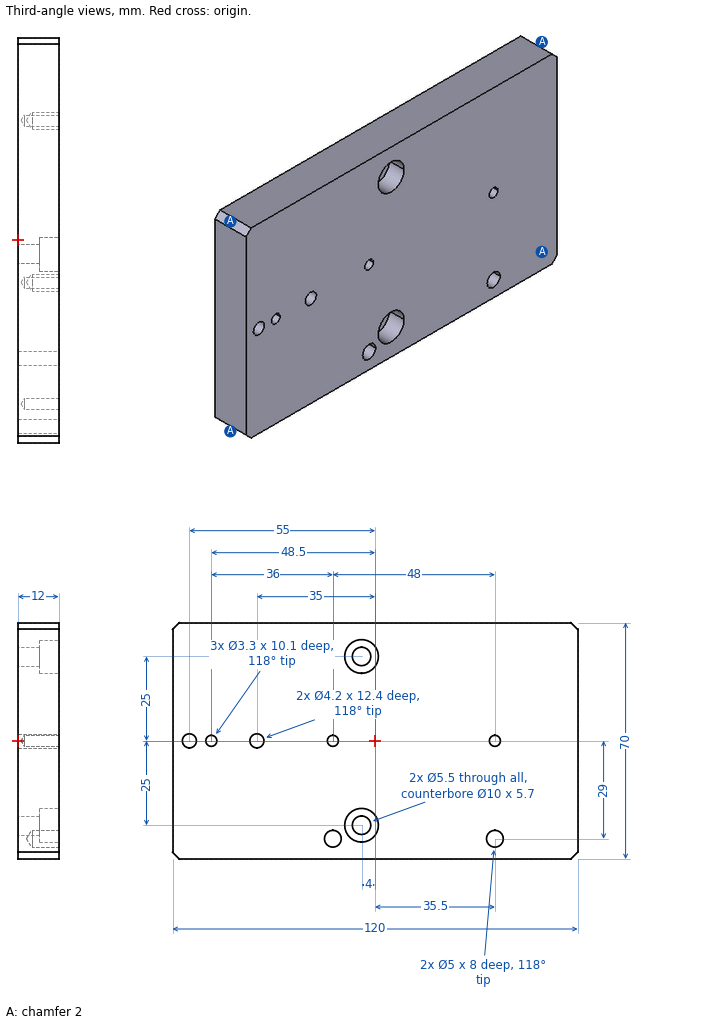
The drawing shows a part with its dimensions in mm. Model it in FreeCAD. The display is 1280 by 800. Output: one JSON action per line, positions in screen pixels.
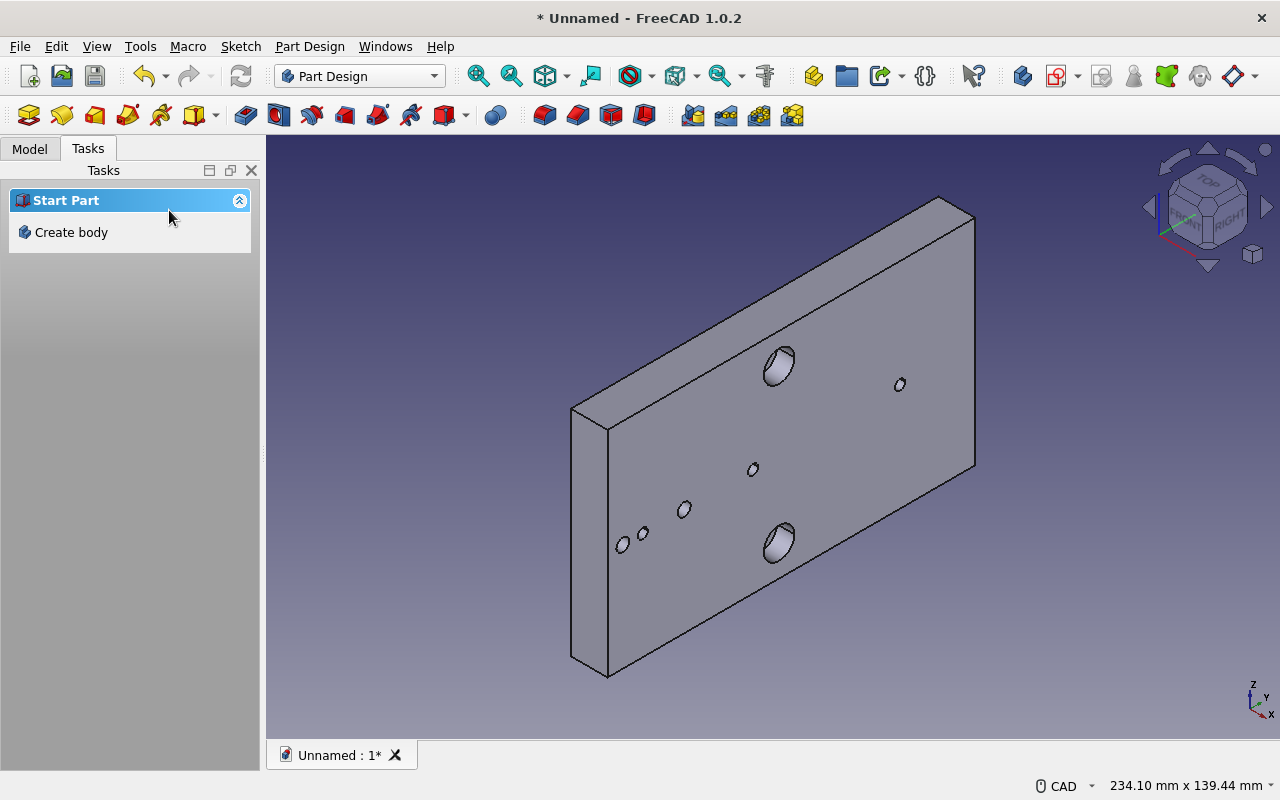
{"action": "left_click", "coordinate": [844, 452]}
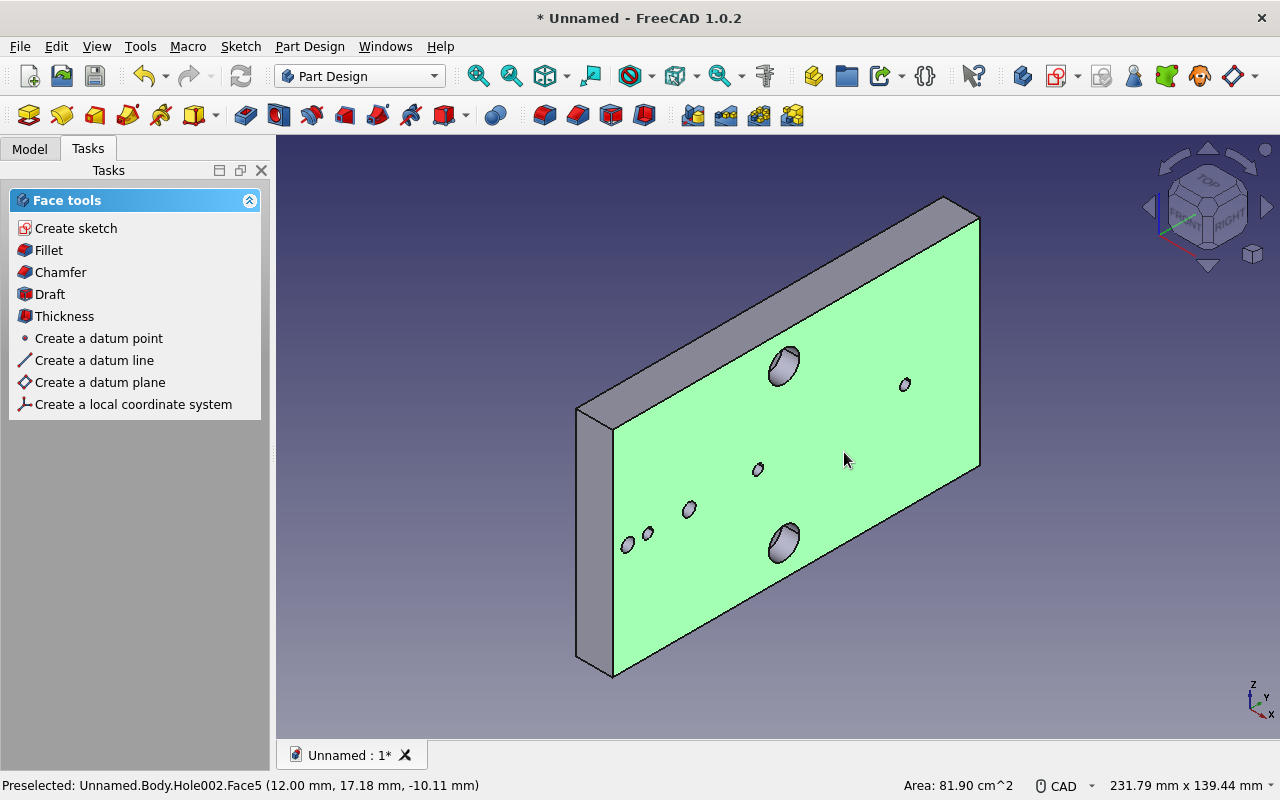
{"action": "left_click", "coordinate": [1056, 76]}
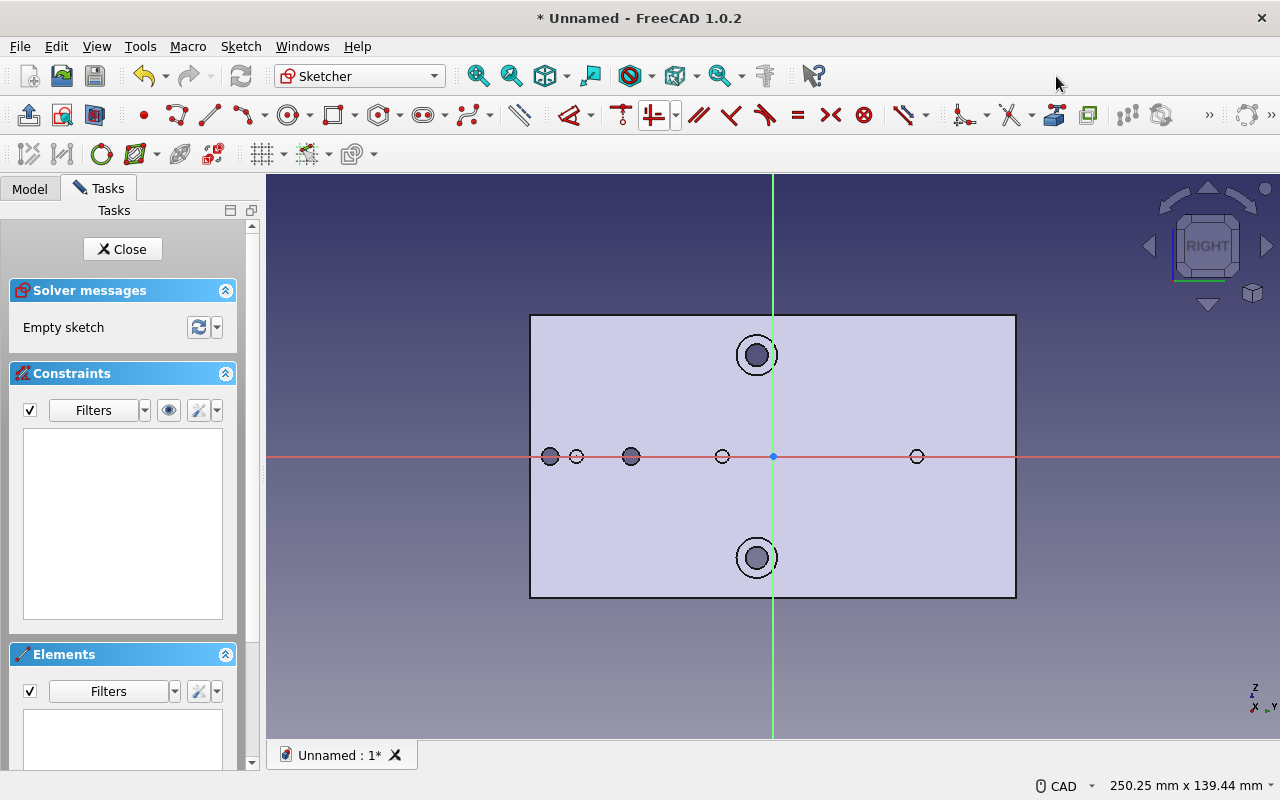
{"action": "scroll", "coordinate": [887, 557], "scroll_direction": "up", "scroll_amount": 5}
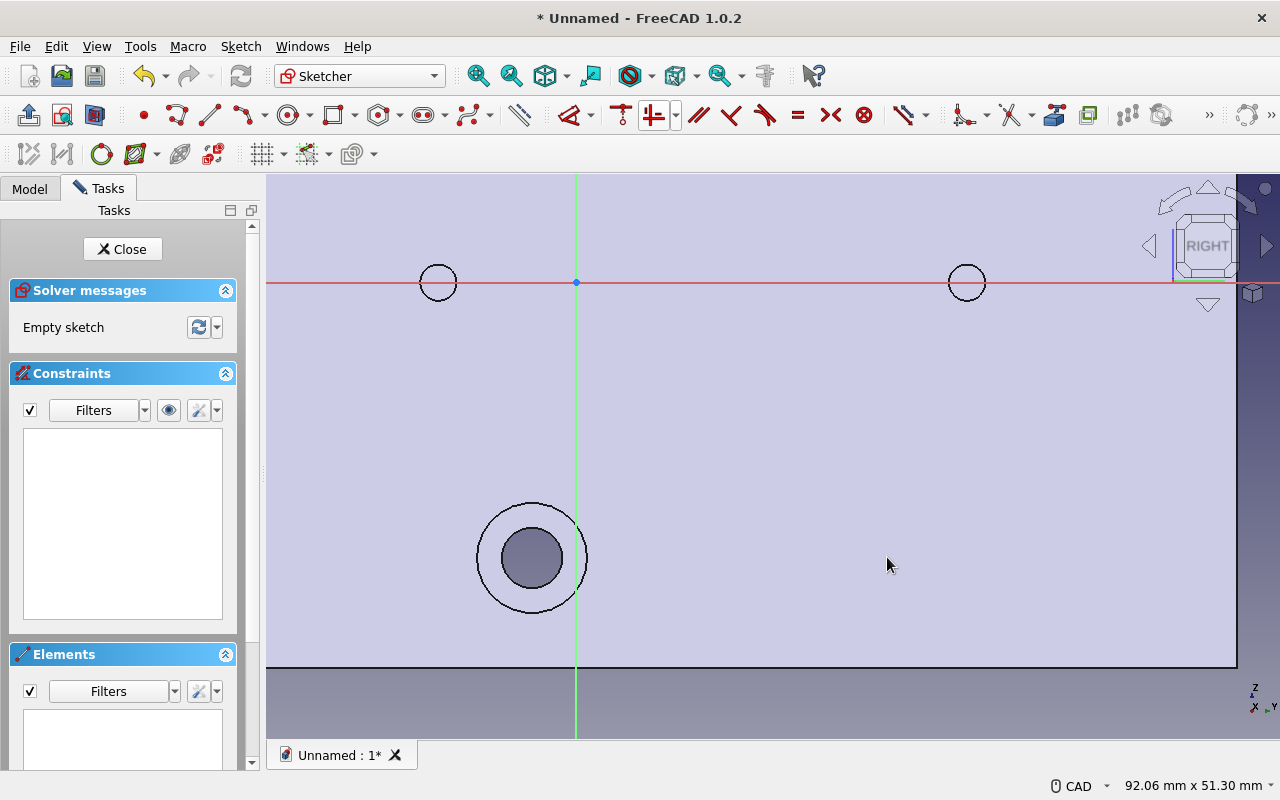
{"action": "left_click", "coordinate": [288, 116]}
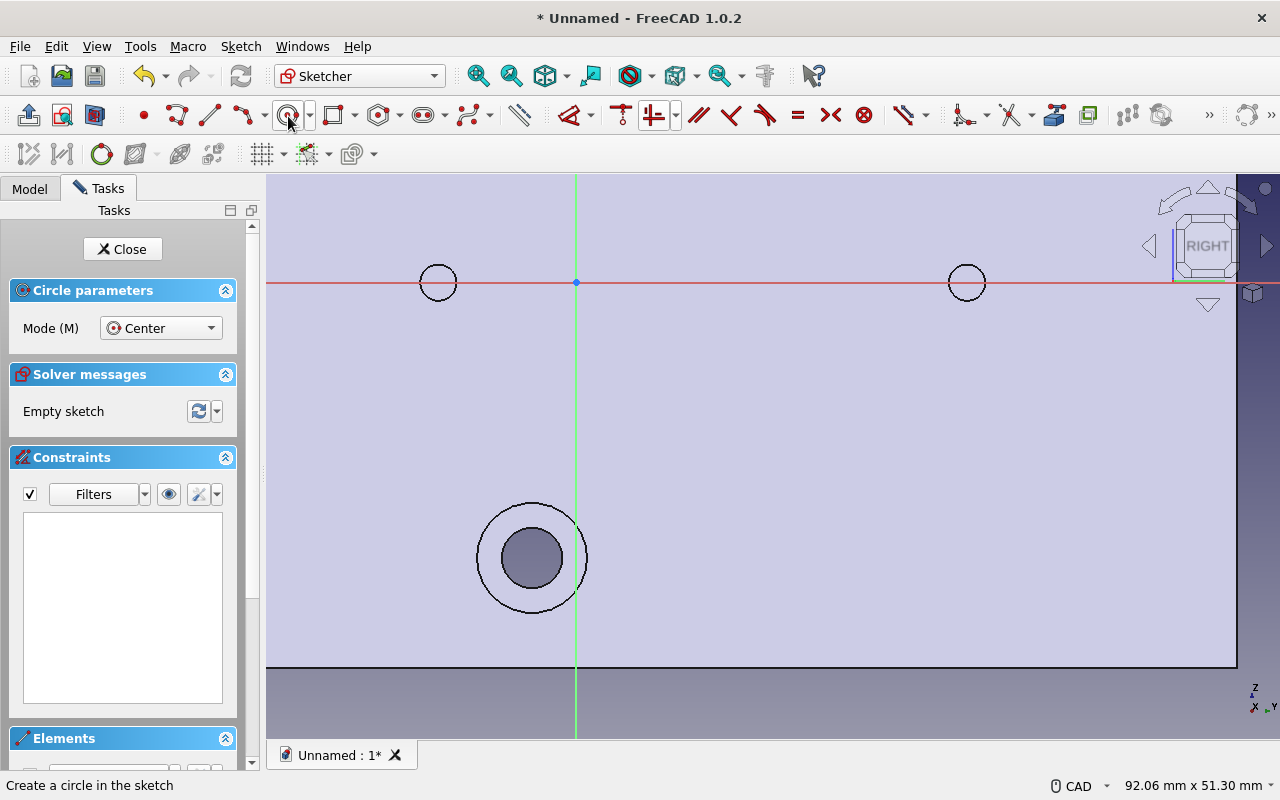
{"action": "left_click", "coordinate": [967, 602]}
{"action": "left_click", "coordinate": [987, 583]}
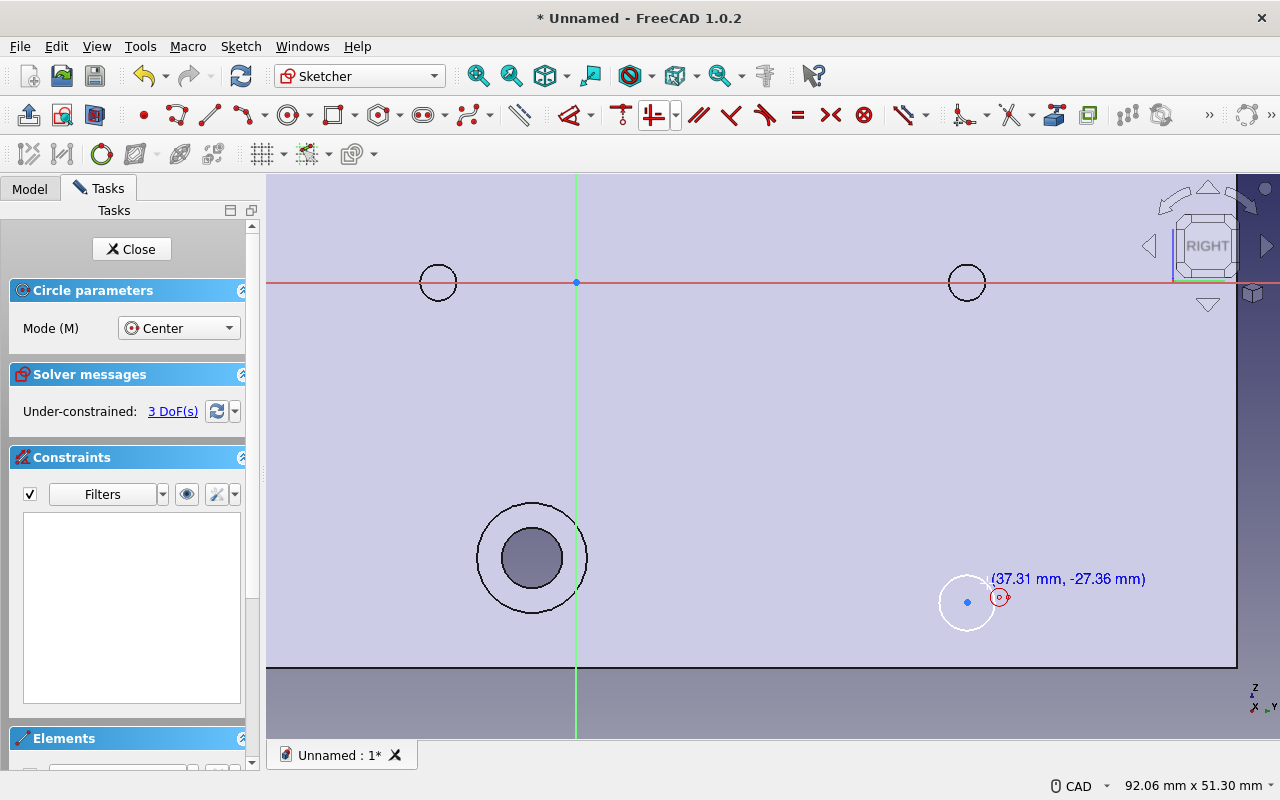
{"action": "left_click", "coordinate": [438, 602]}
{"action": "left_click", "coordinate": [458, 583]}
{"action": "key", "text": "Escape"}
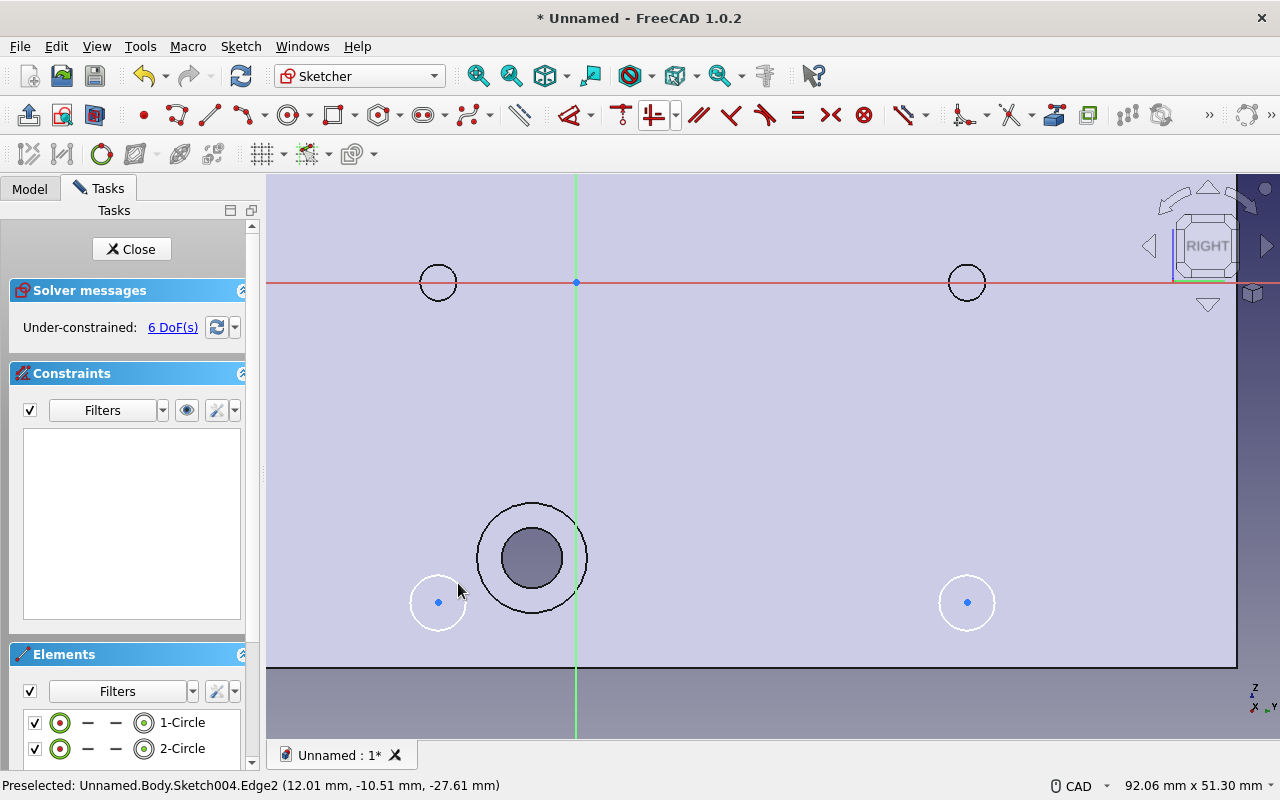
{"action": "left_click", "coordinate": [986, 583]}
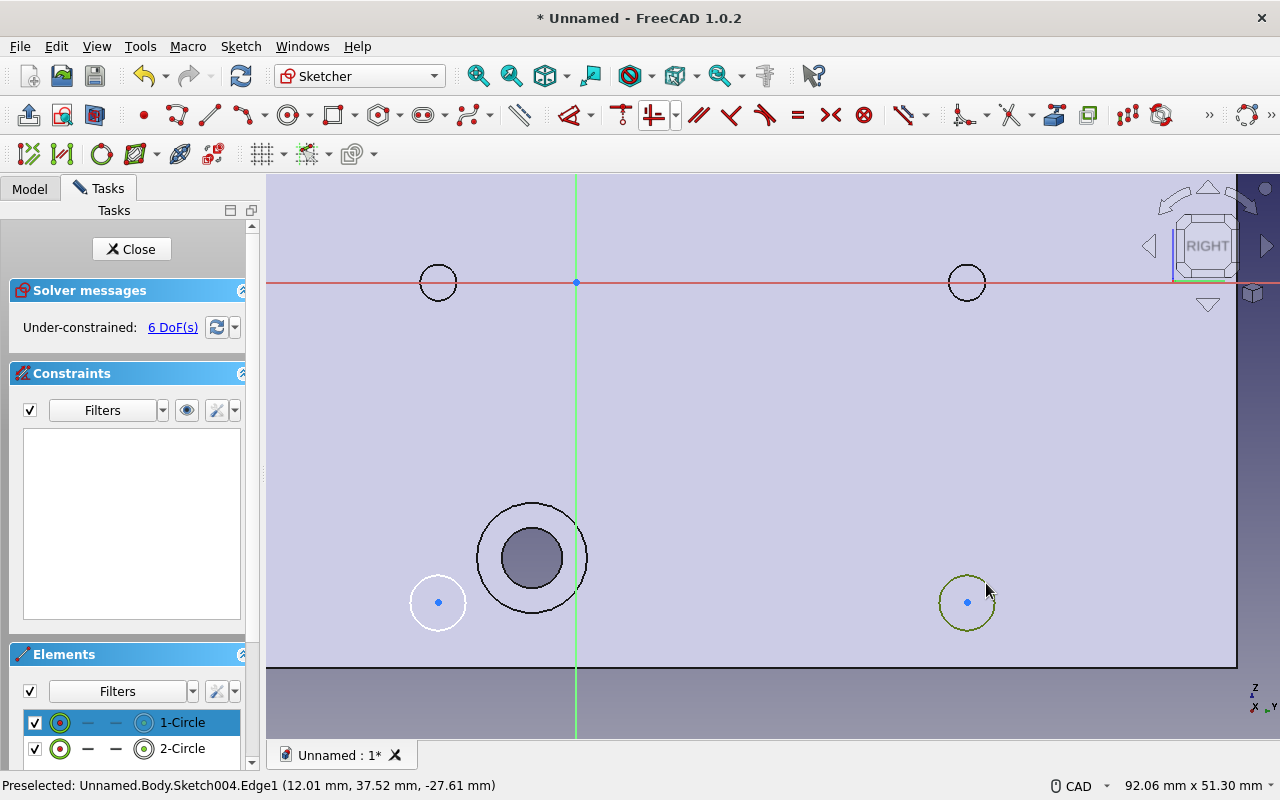
{"action": "left_click", "coordinate": [457, 583]}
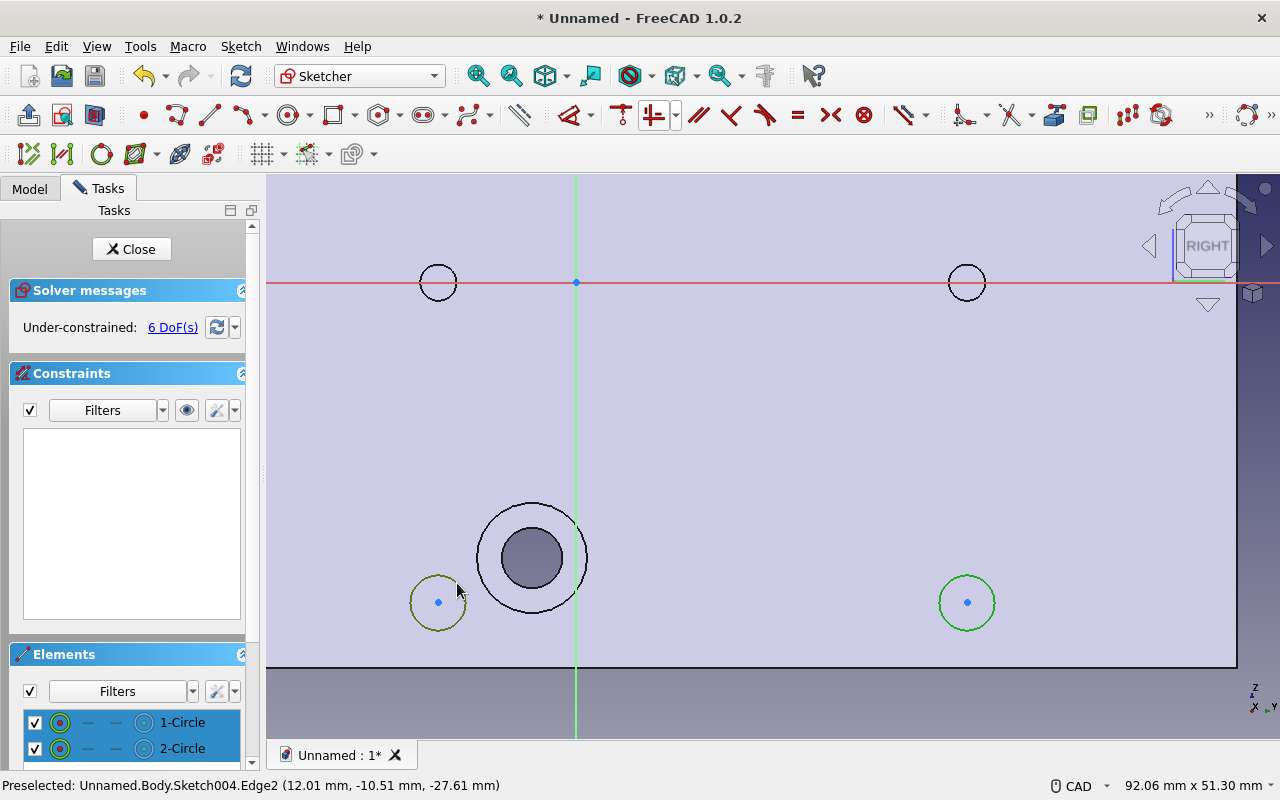
{"action": "key", "text": "e"}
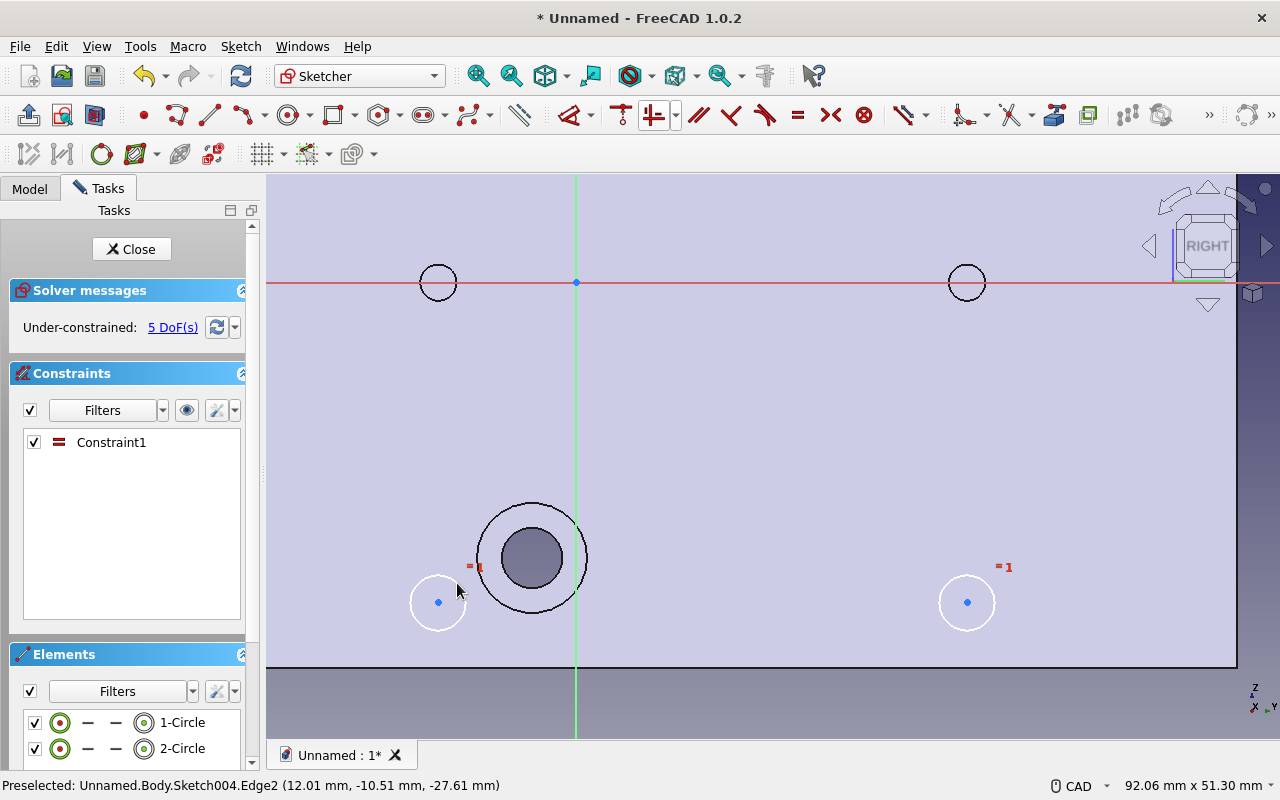
{"action": "left_click", "coordinate": [967, 603]}